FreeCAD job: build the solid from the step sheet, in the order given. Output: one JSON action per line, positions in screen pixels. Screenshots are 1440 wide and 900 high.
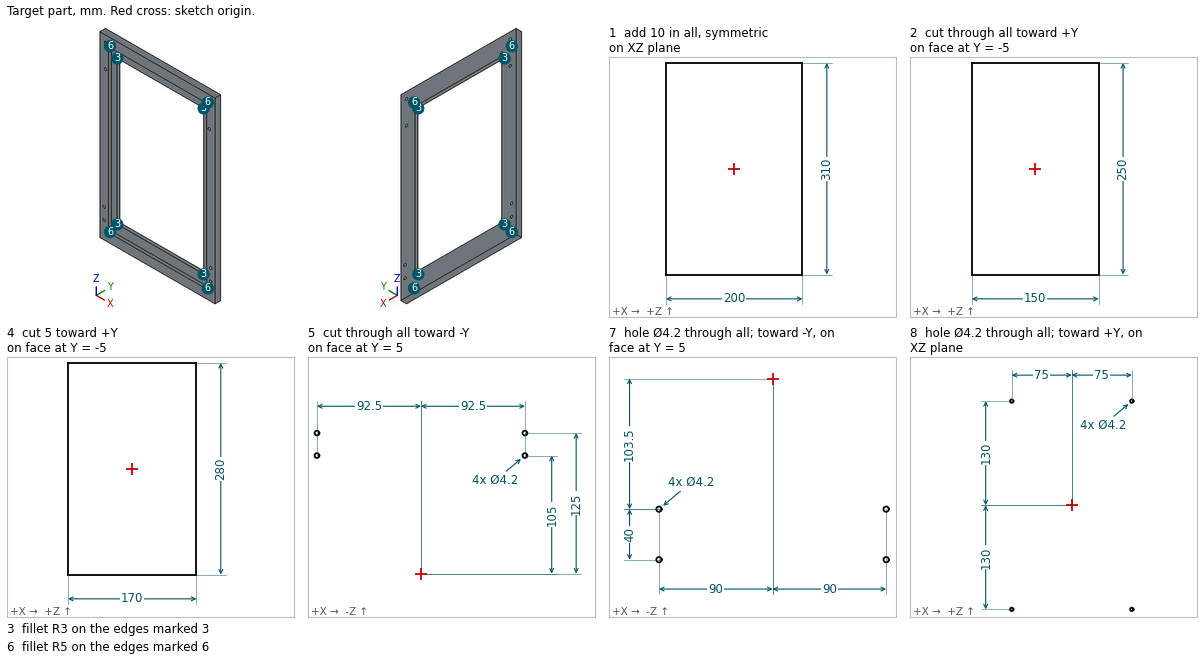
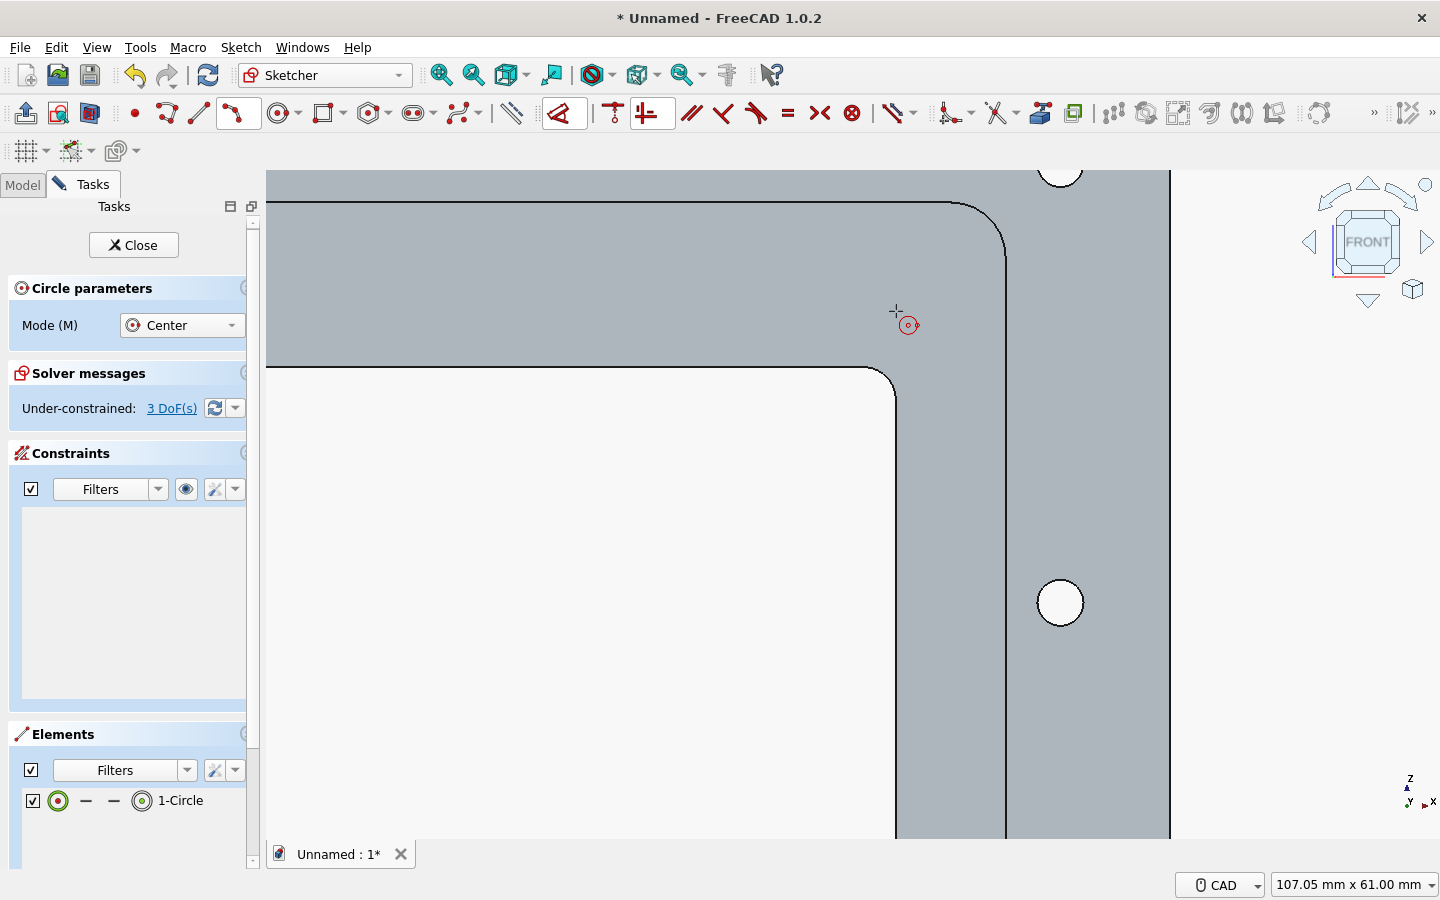
{"action": "scroll", "coordinate": [896, 311], "scroll_direction": "down", "scroll_amount": 10}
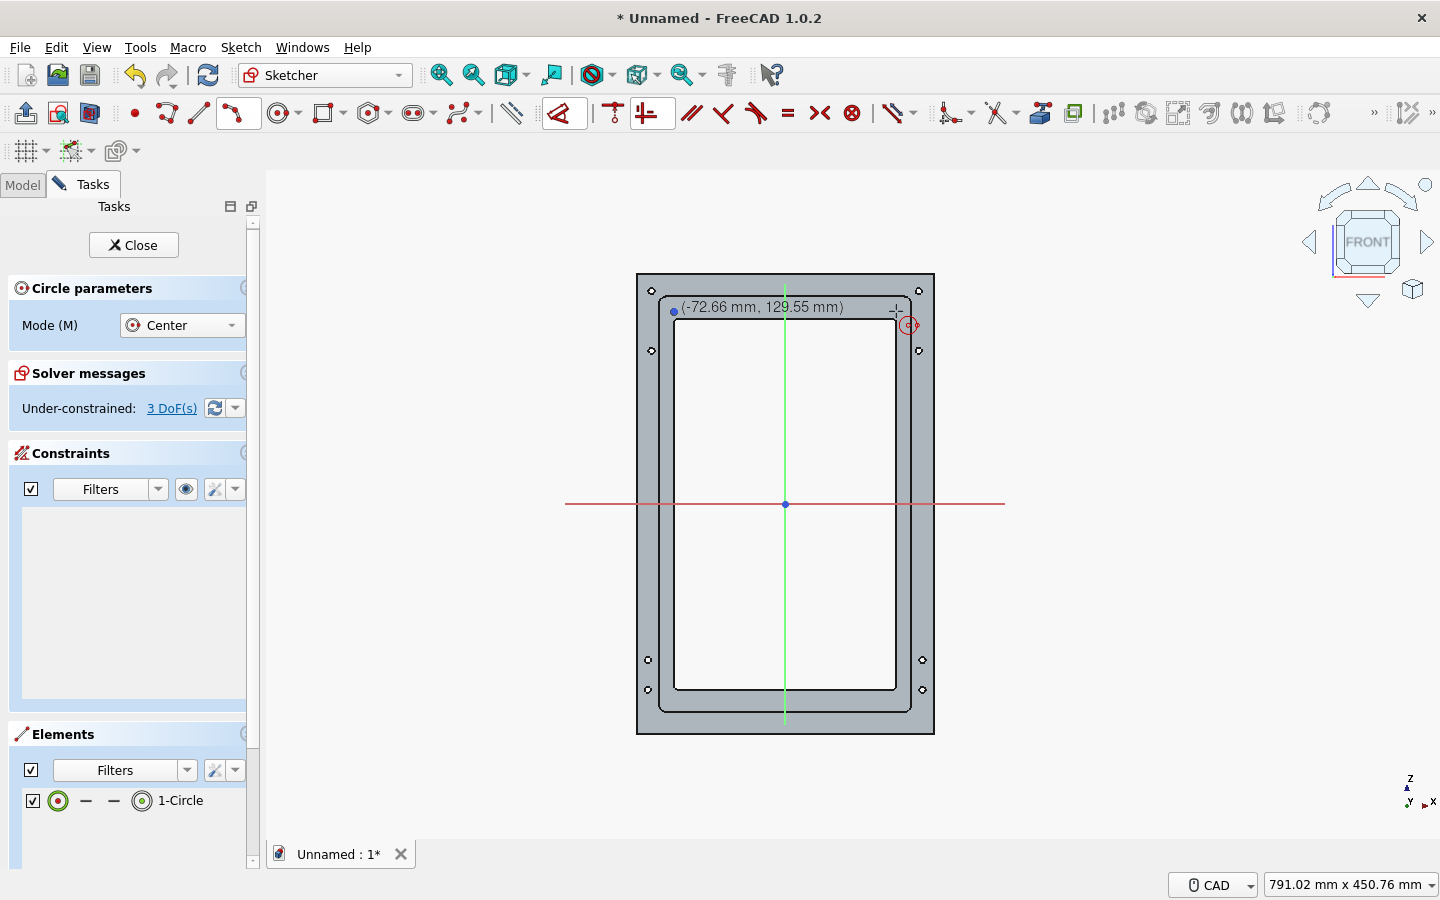
{"action": "left_click", "coordinate": [896, 311]}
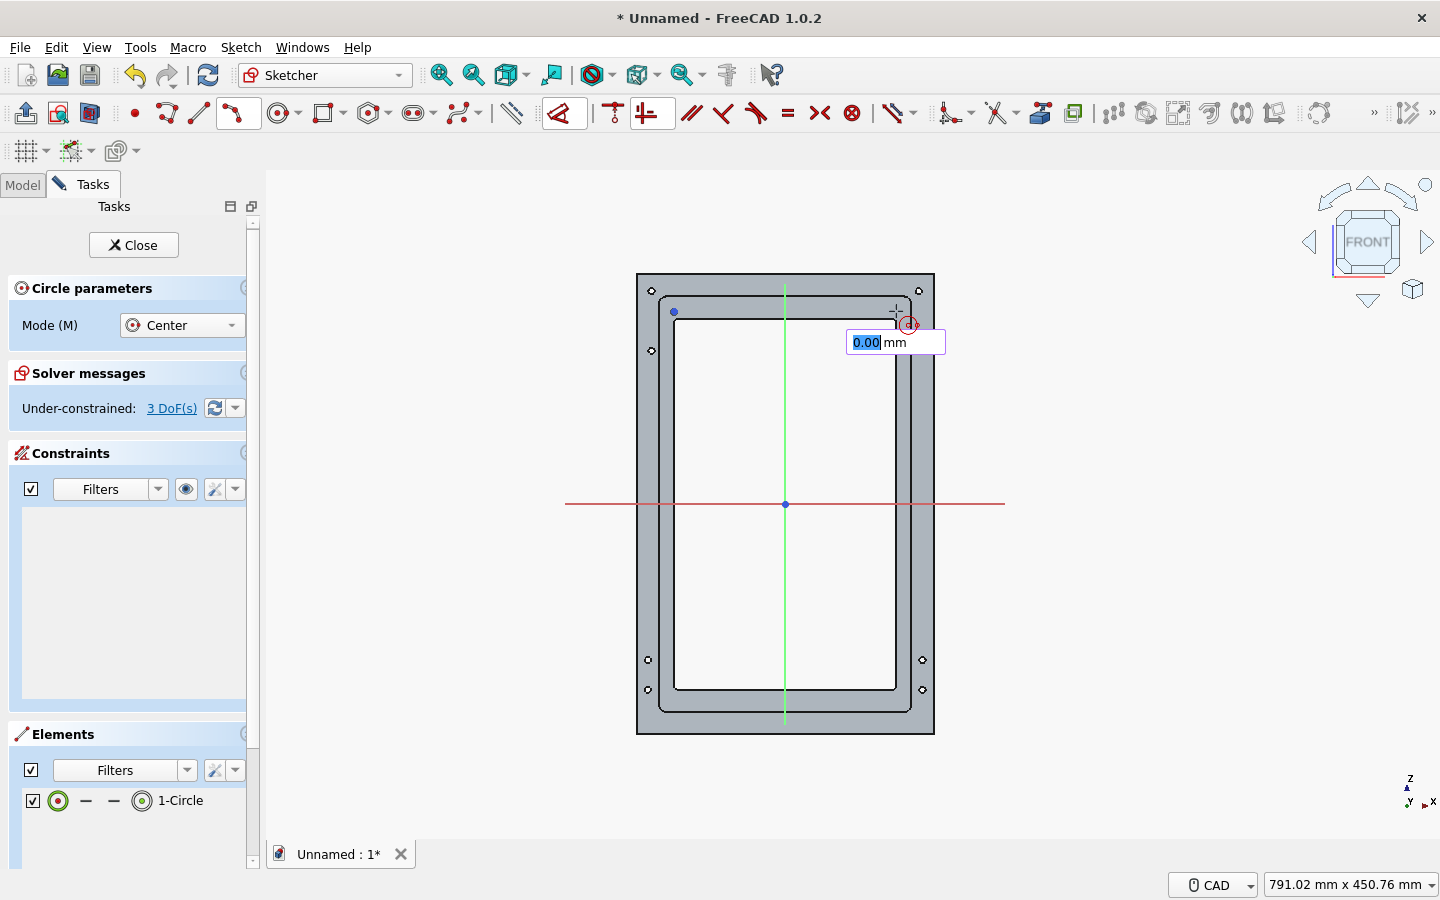
{"action": "scroll", "coordinate": [899, 309], "scroll_direction": "up", "scroll_amount": 9}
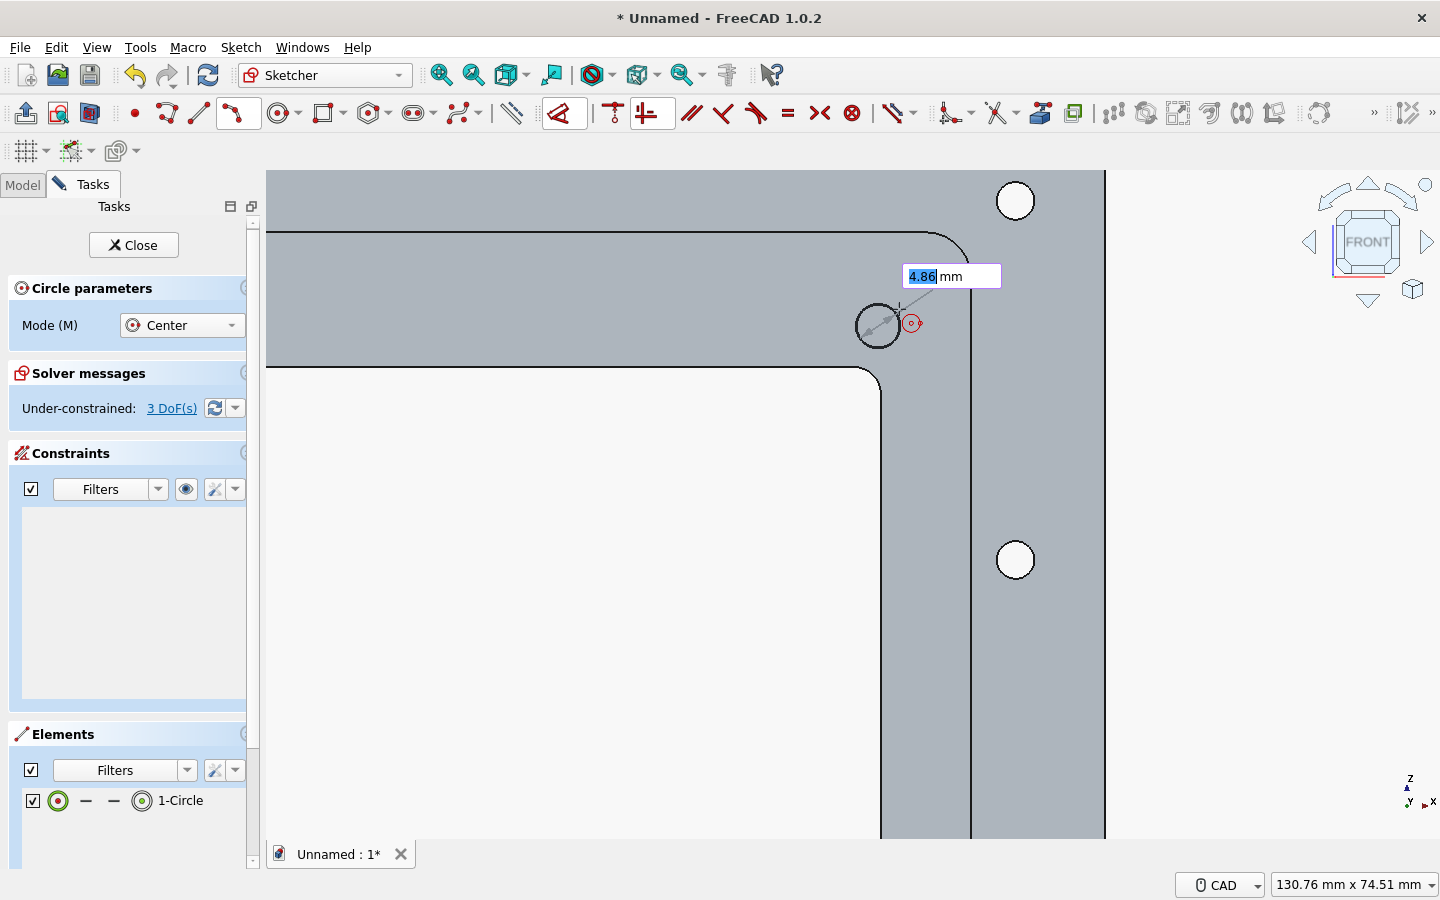
{"action": "left_click", "coordinate": [894, 309]}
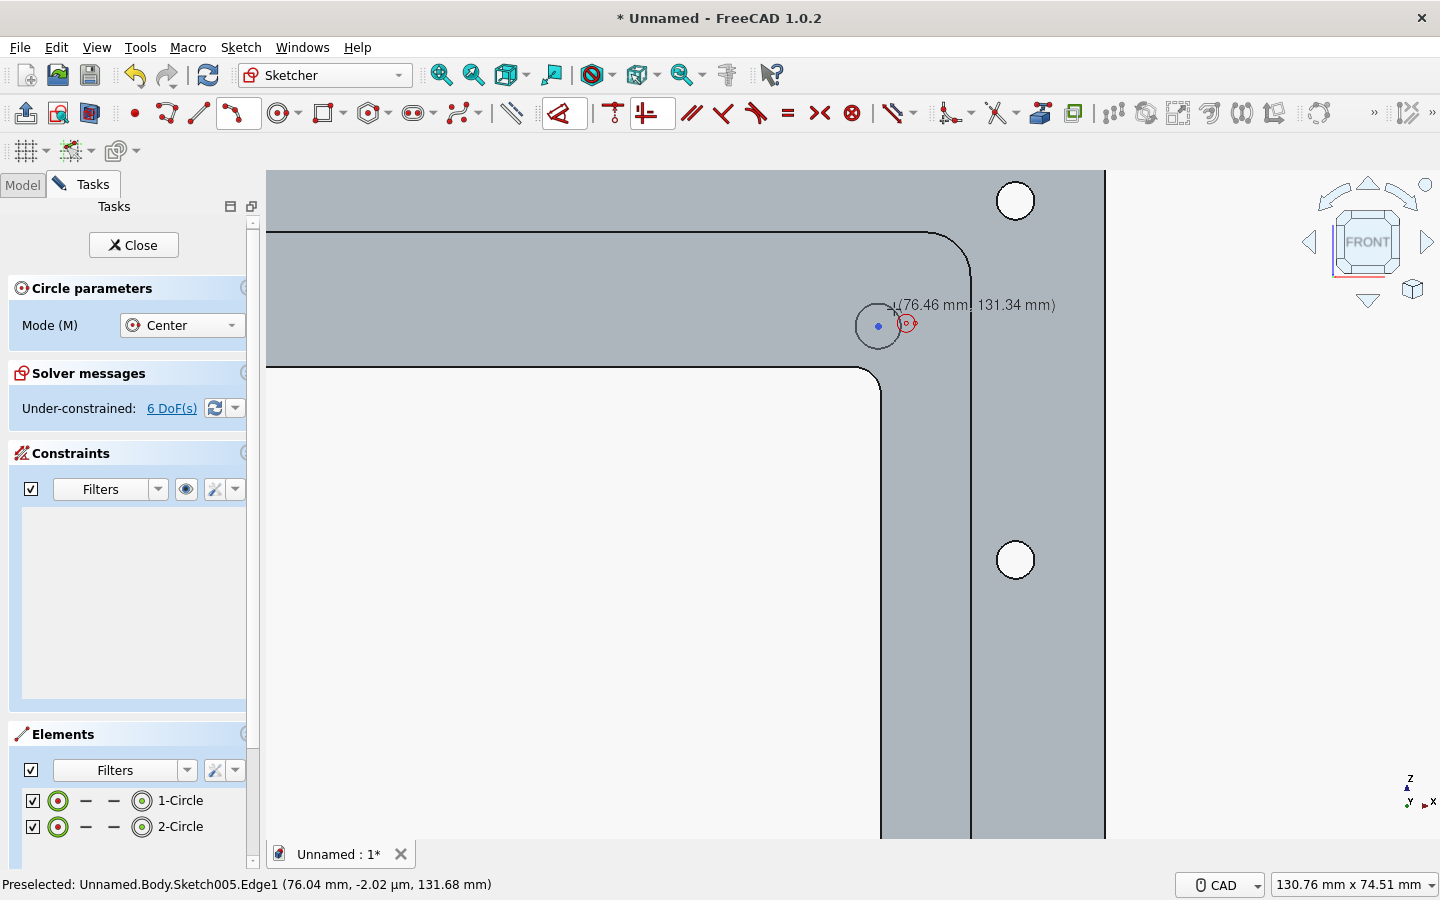
{"action": "scroll", "coordinate": [899, 309], "scroll_direction": "down", "scroll_amount": 9}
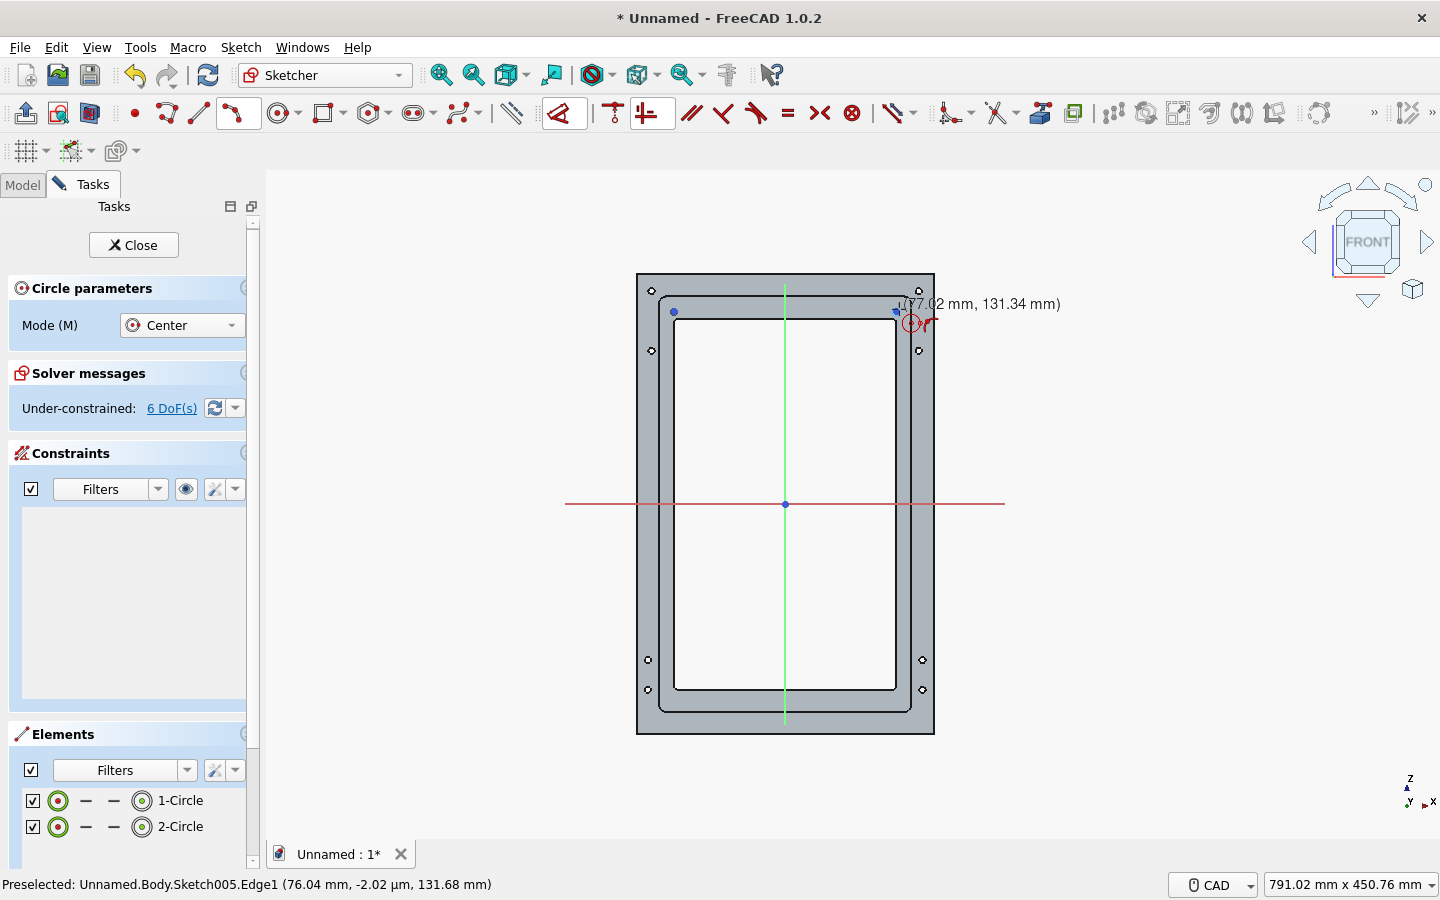
{"action": "scroll", "coordinate": [674, 697], "scroll_direction": "up", "scroll_amount": 10}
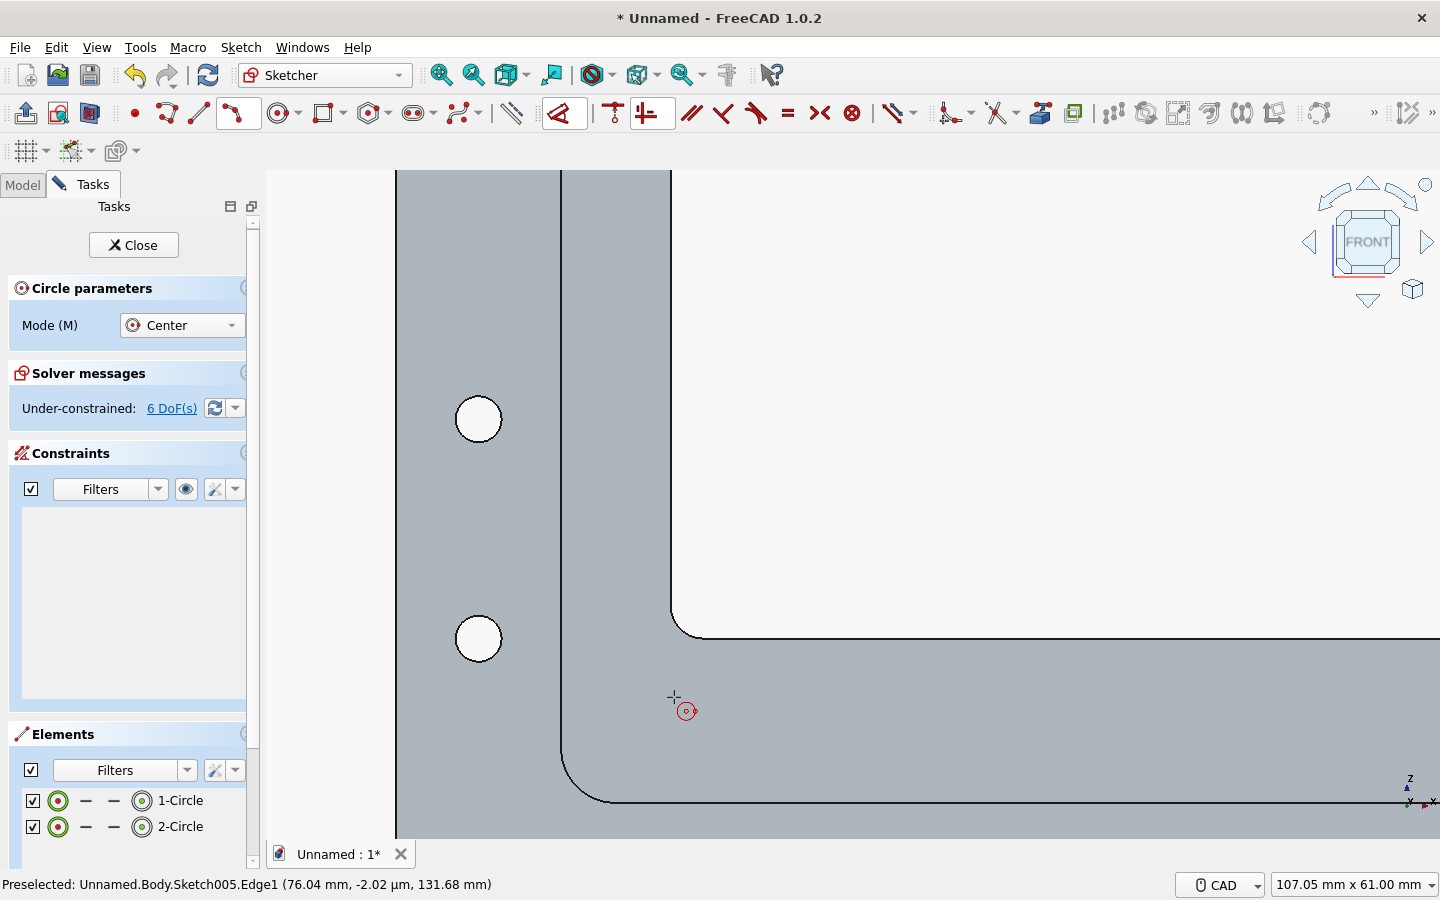
{"action": "scroll", "coordinate": [674, 698], "scroll_direction": "down", "scroll_amount": 10}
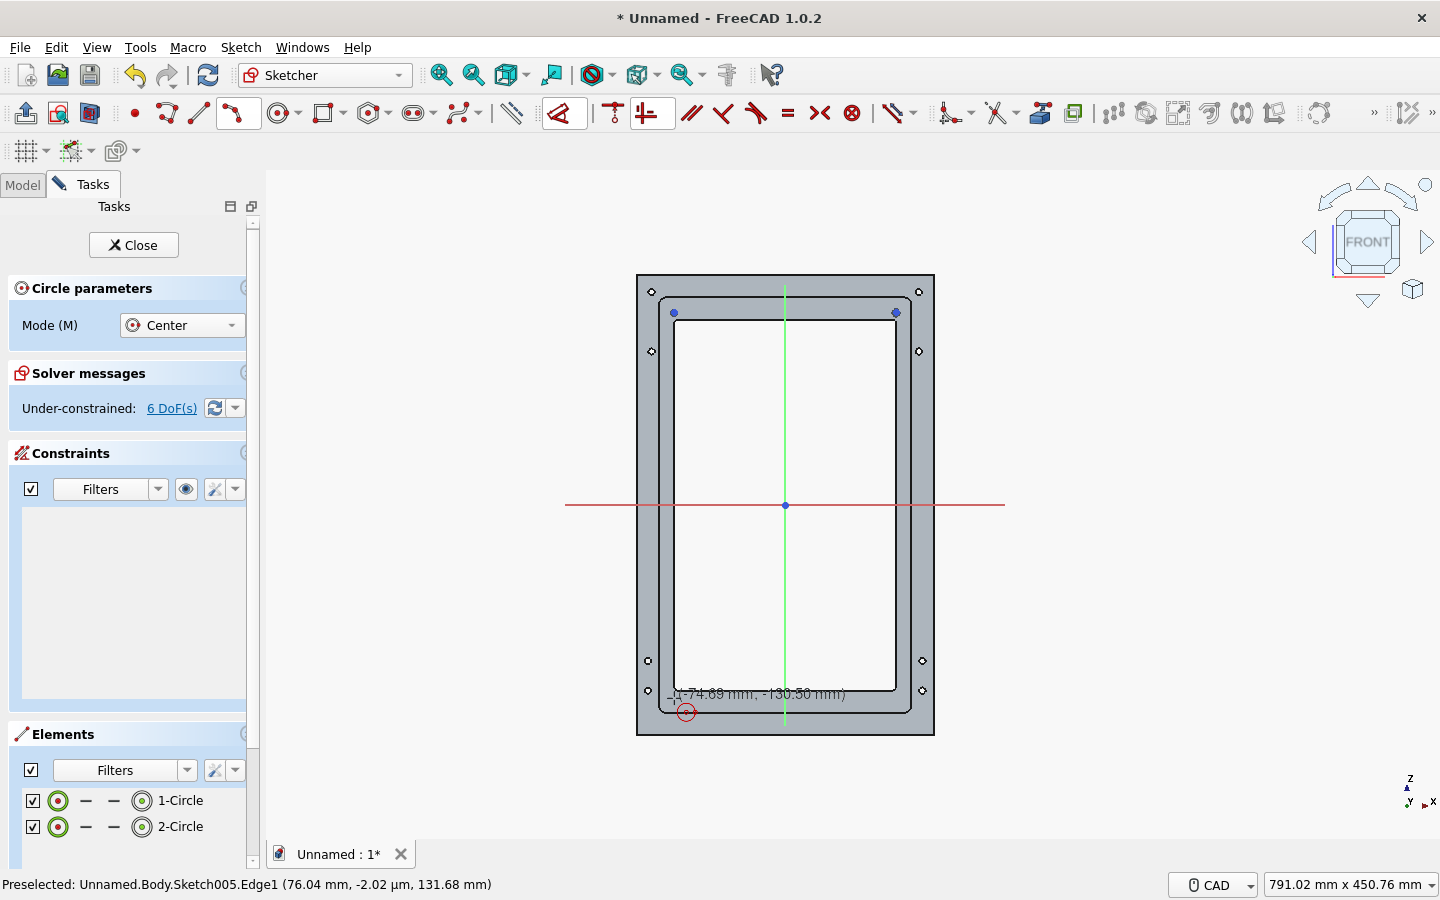
{"action": "left_click", "coordinate": [674, 698]}